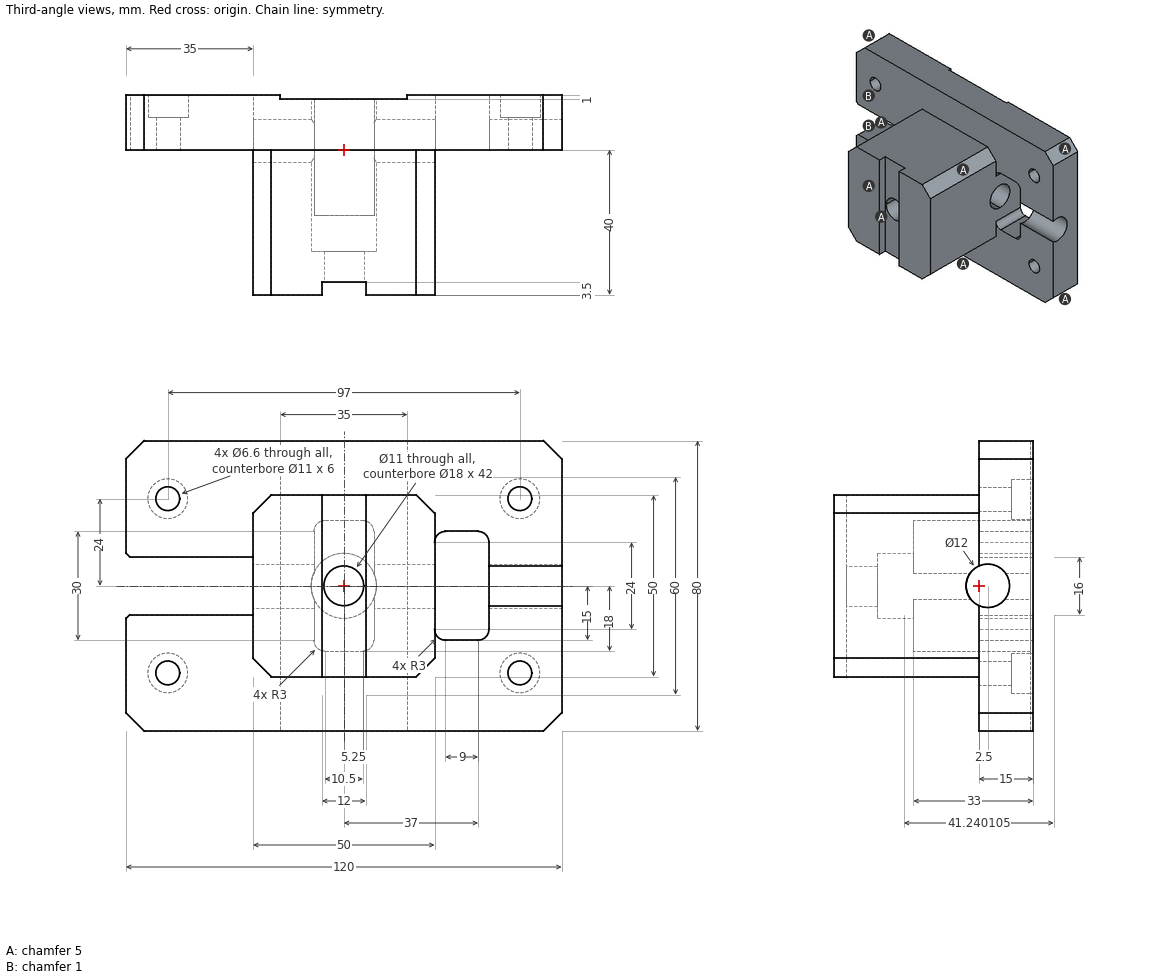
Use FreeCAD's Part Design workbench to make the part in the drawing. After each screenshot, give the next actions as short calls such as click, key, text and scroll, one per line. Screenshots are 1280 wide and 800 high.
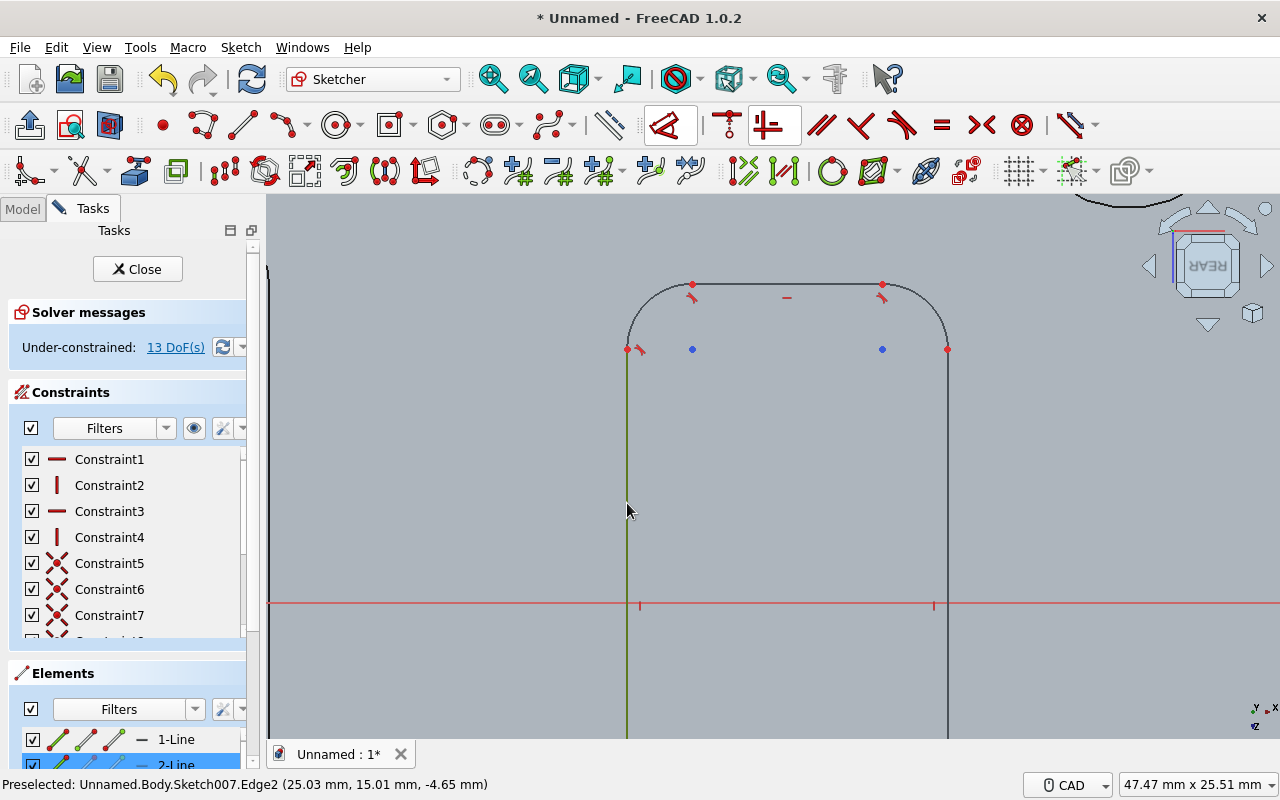
scroll(929, 300, down, 3)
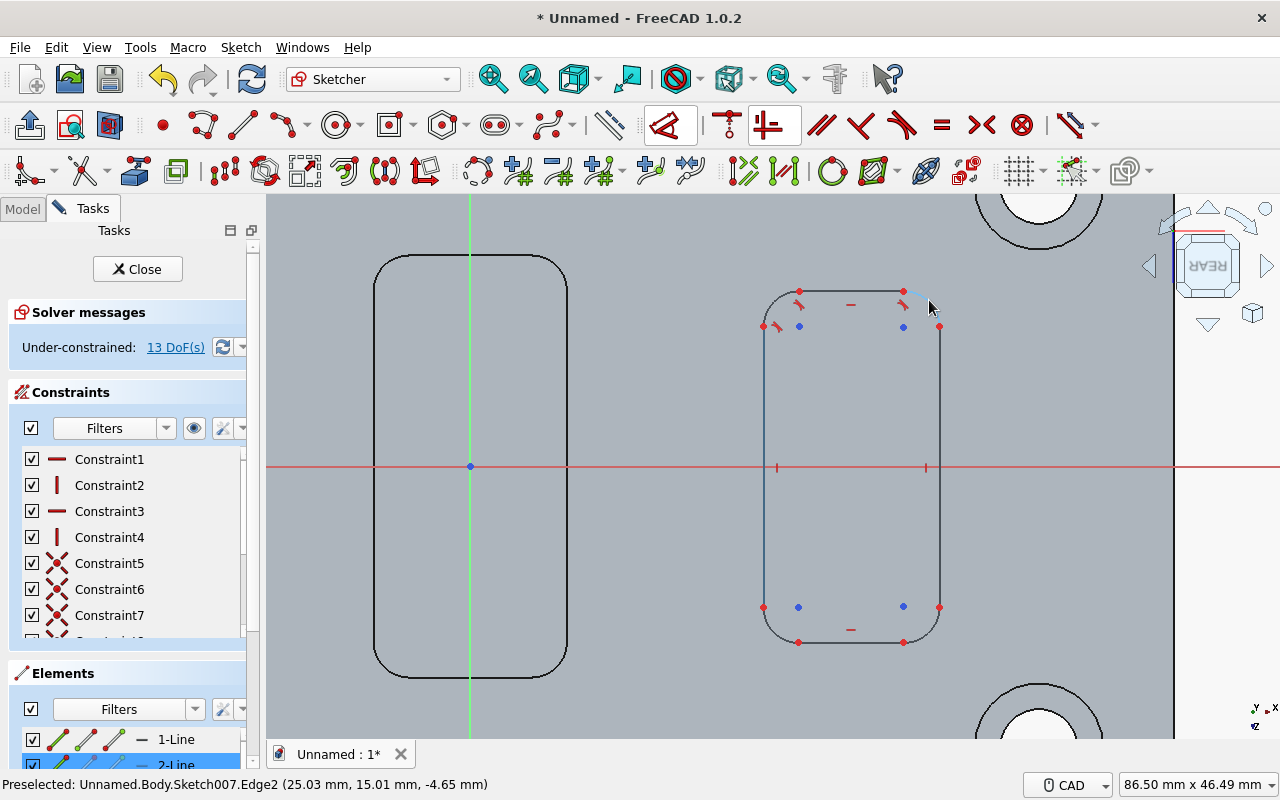
click(768, 624)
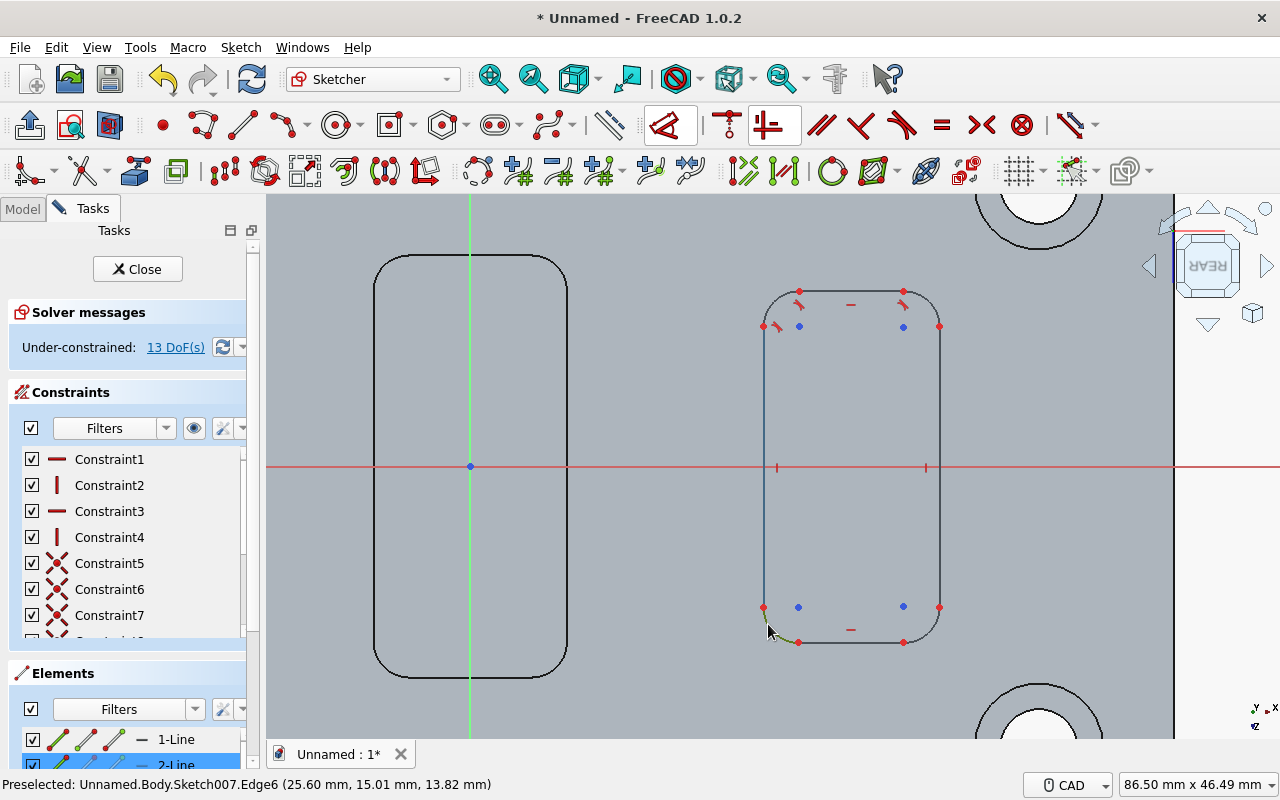
click(902, 126)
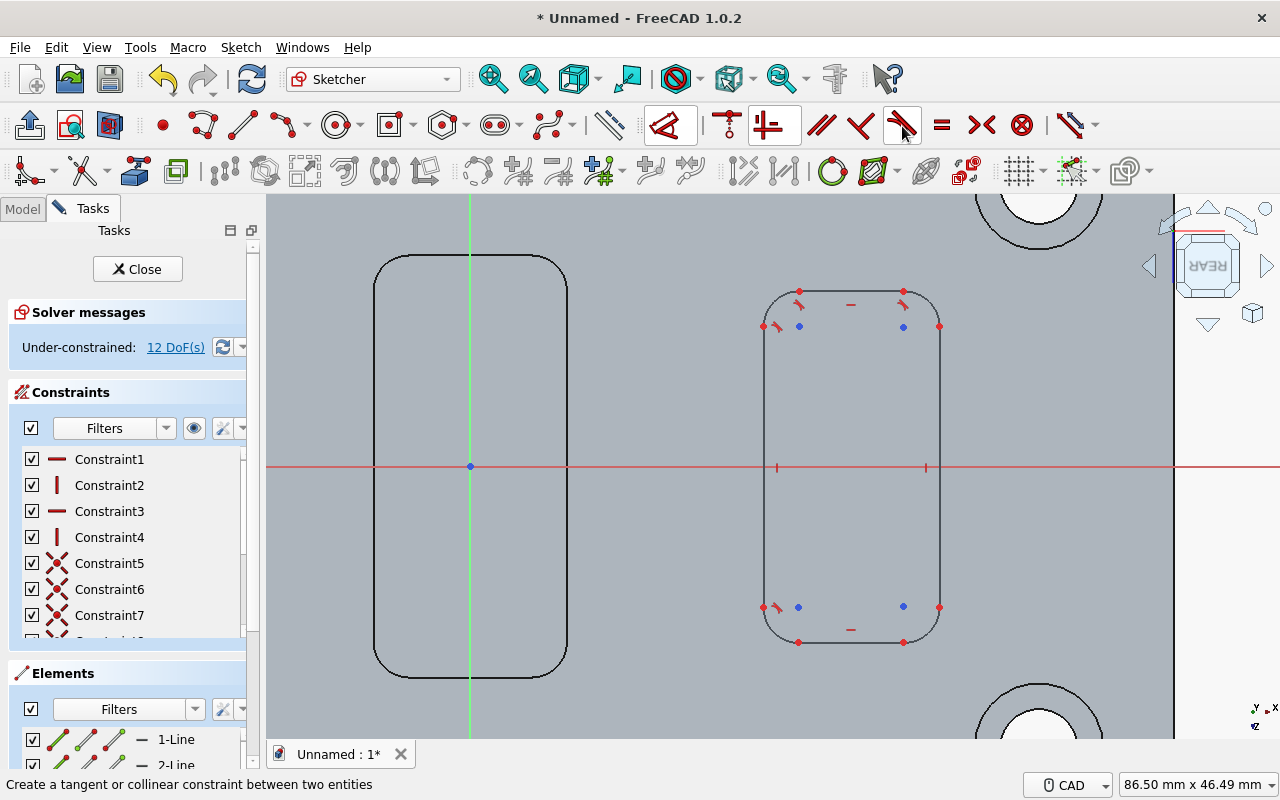
click(830, 643)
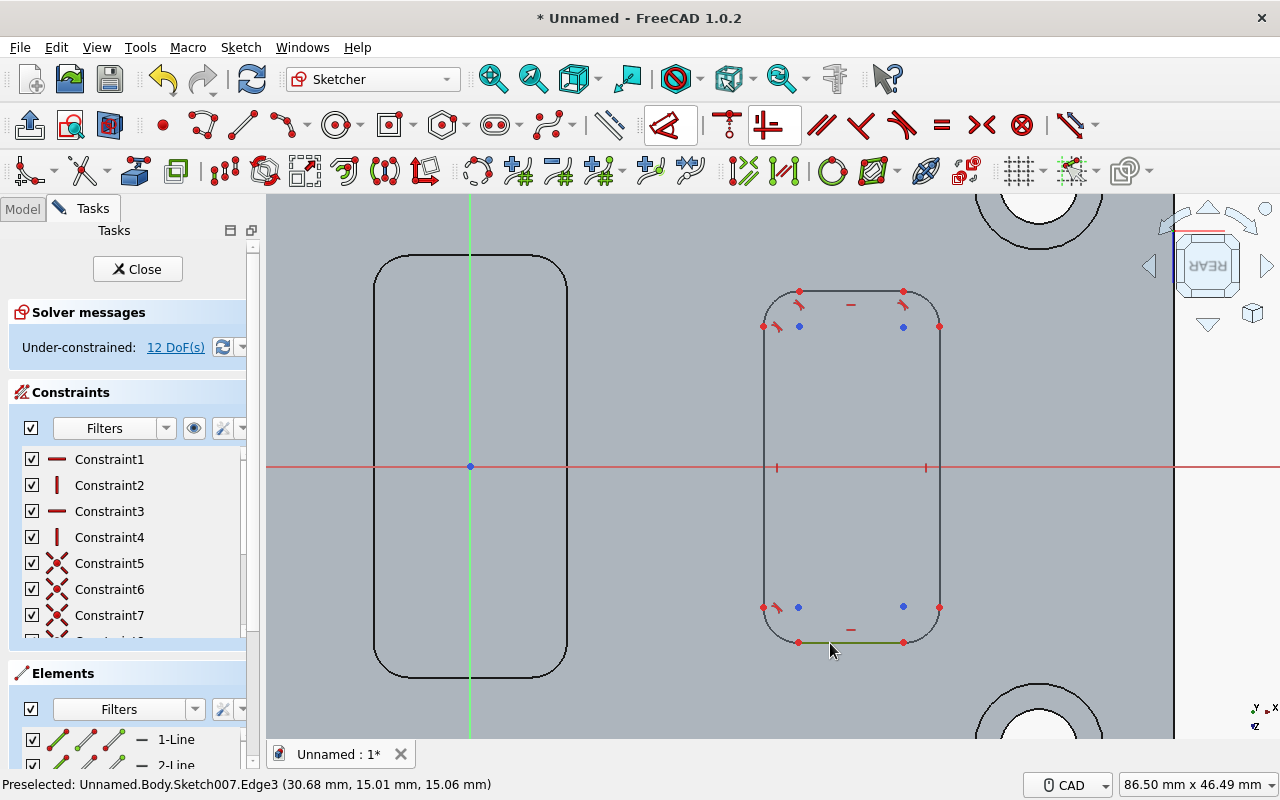
click(768, 624)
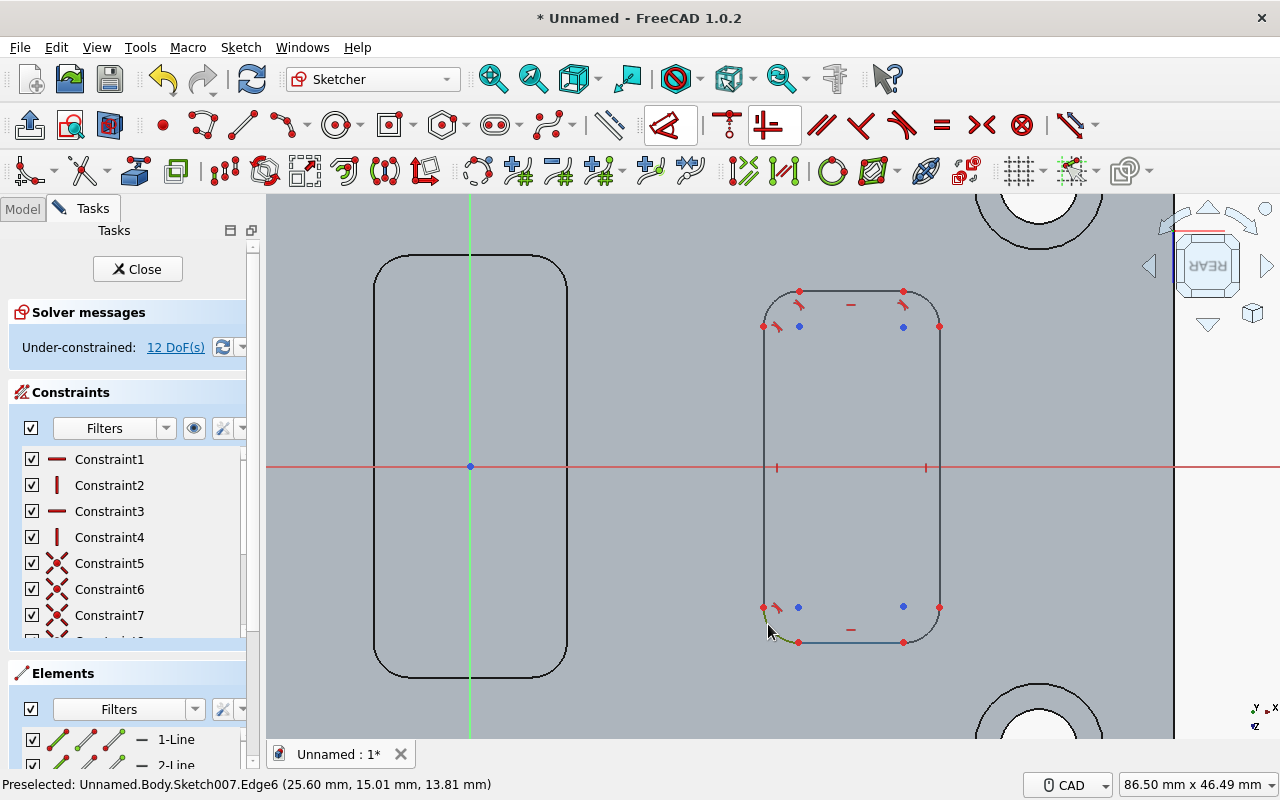
click(902, 126)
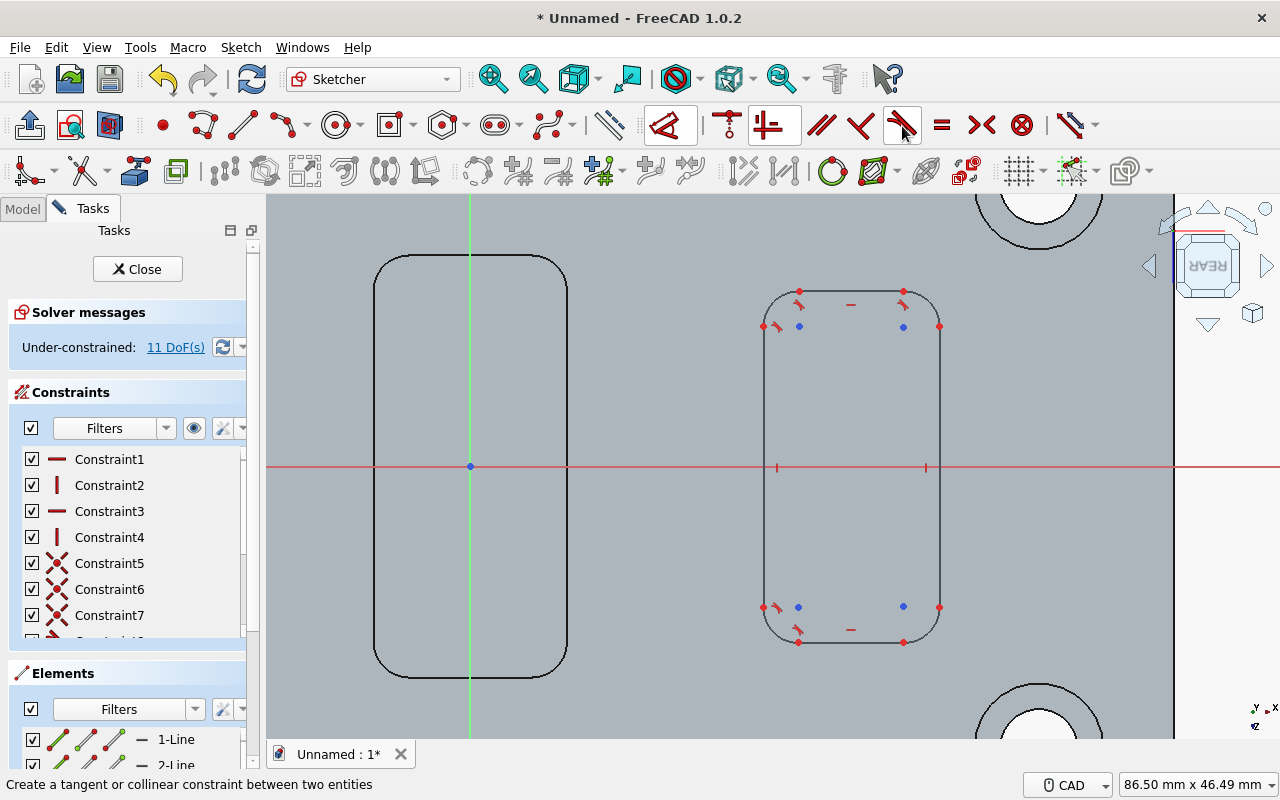
click(830, 643)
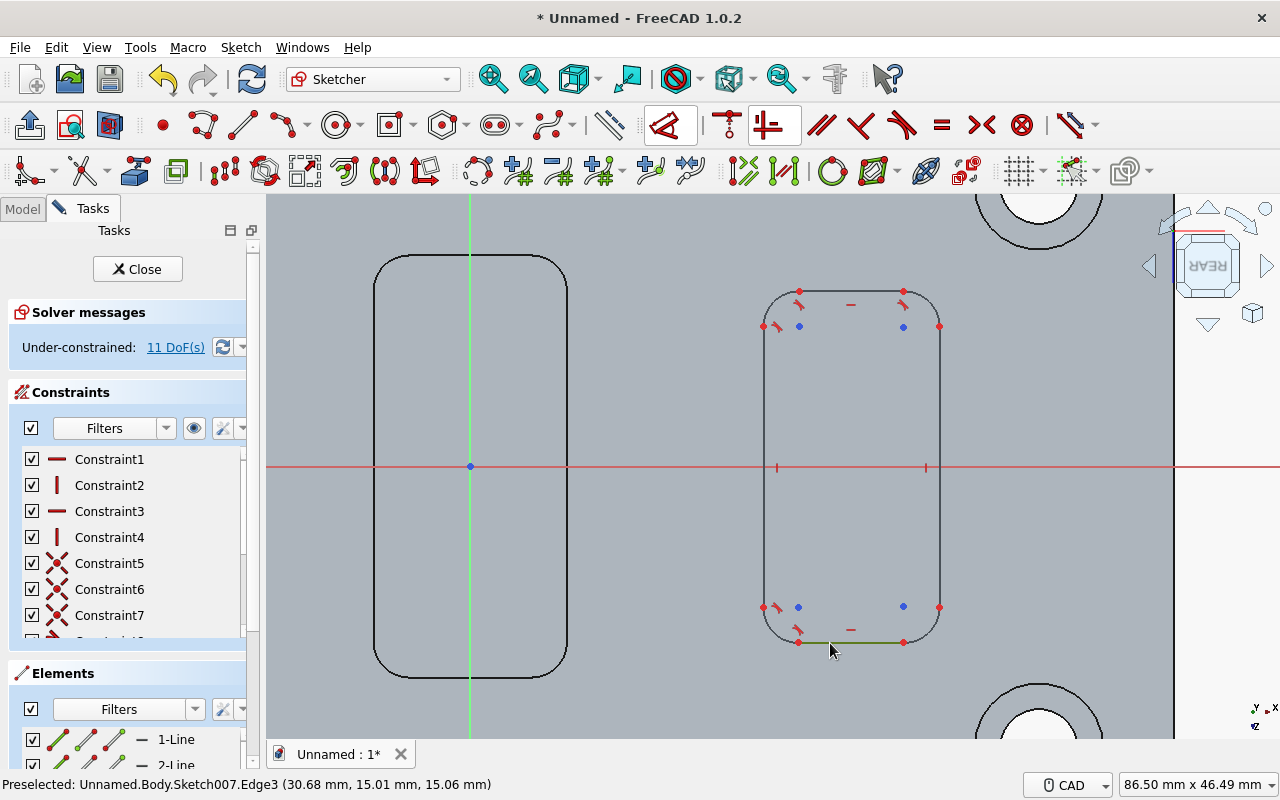
click(920, 639)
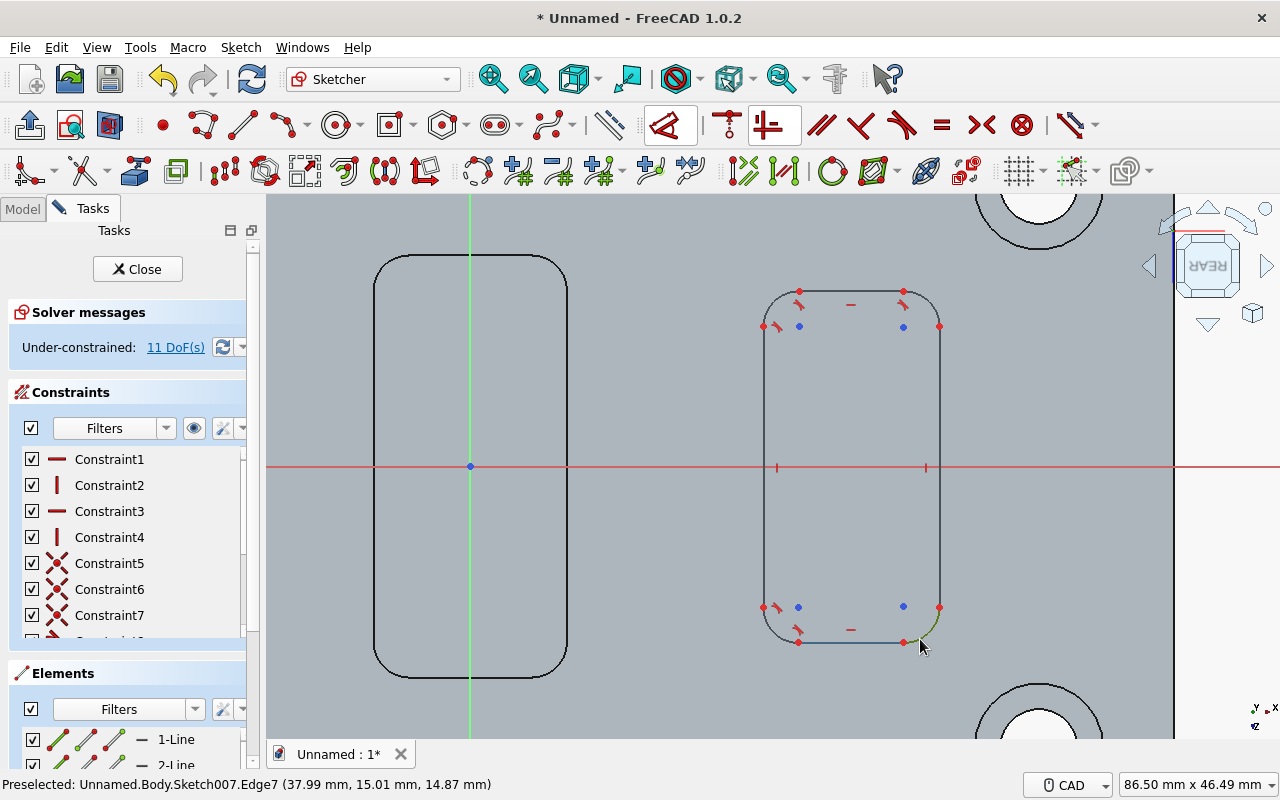
key(t)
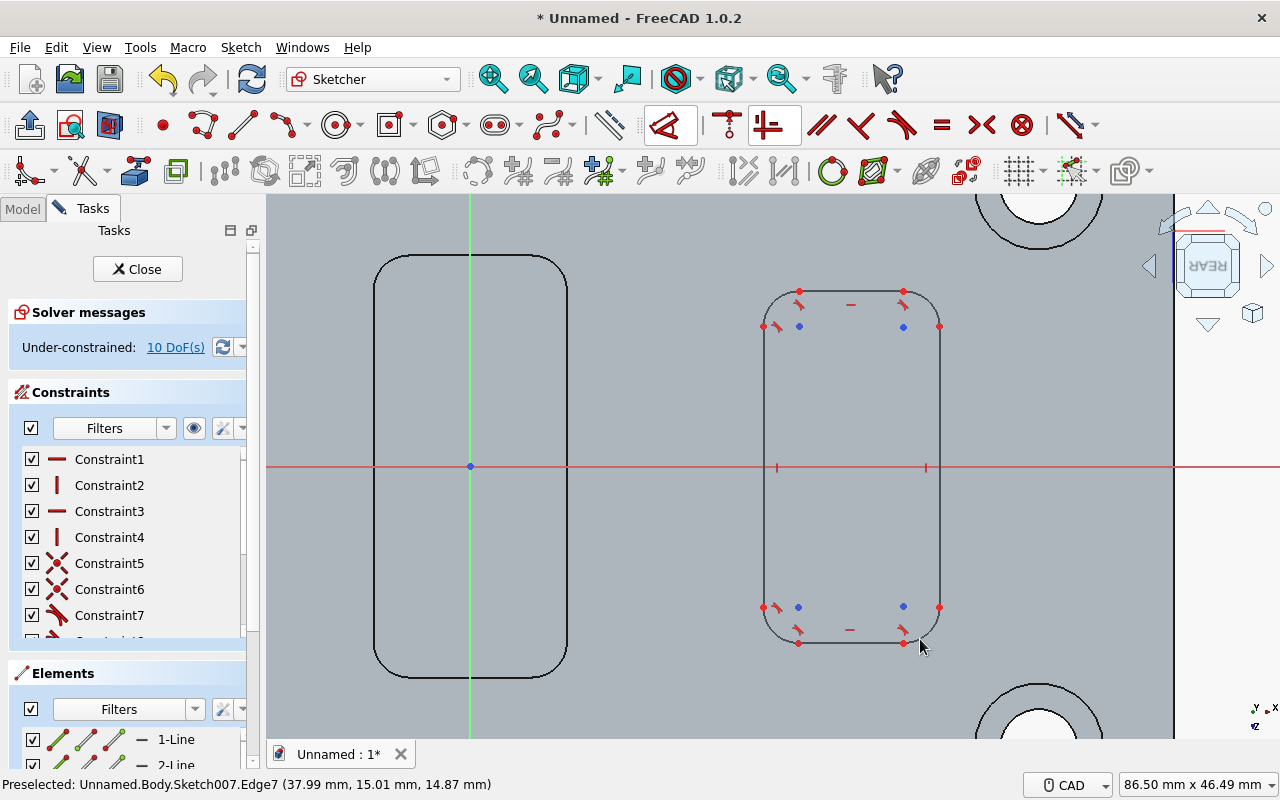
click(940, 524)